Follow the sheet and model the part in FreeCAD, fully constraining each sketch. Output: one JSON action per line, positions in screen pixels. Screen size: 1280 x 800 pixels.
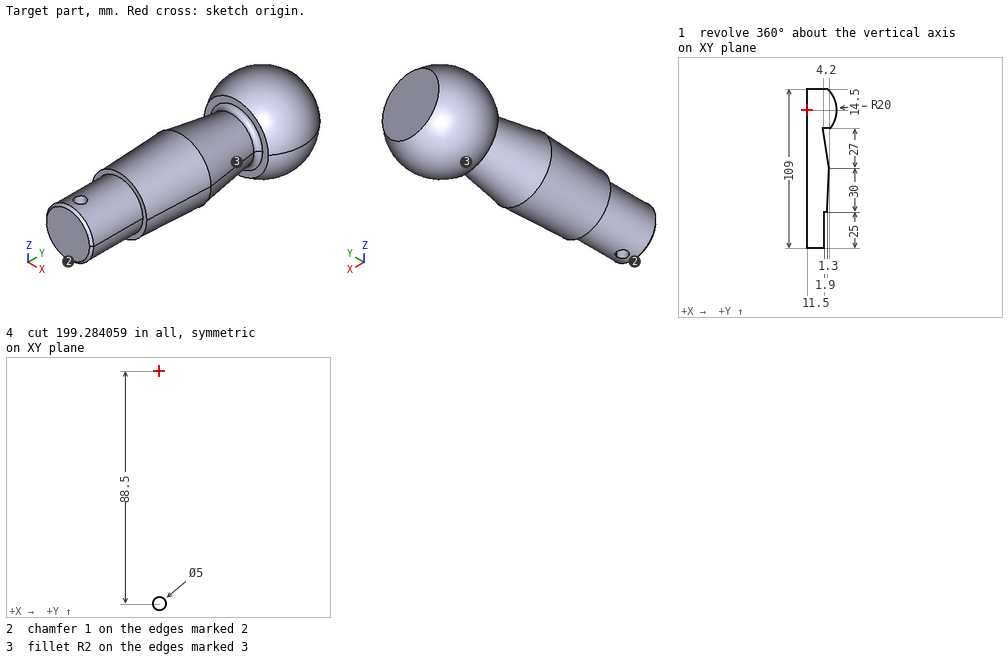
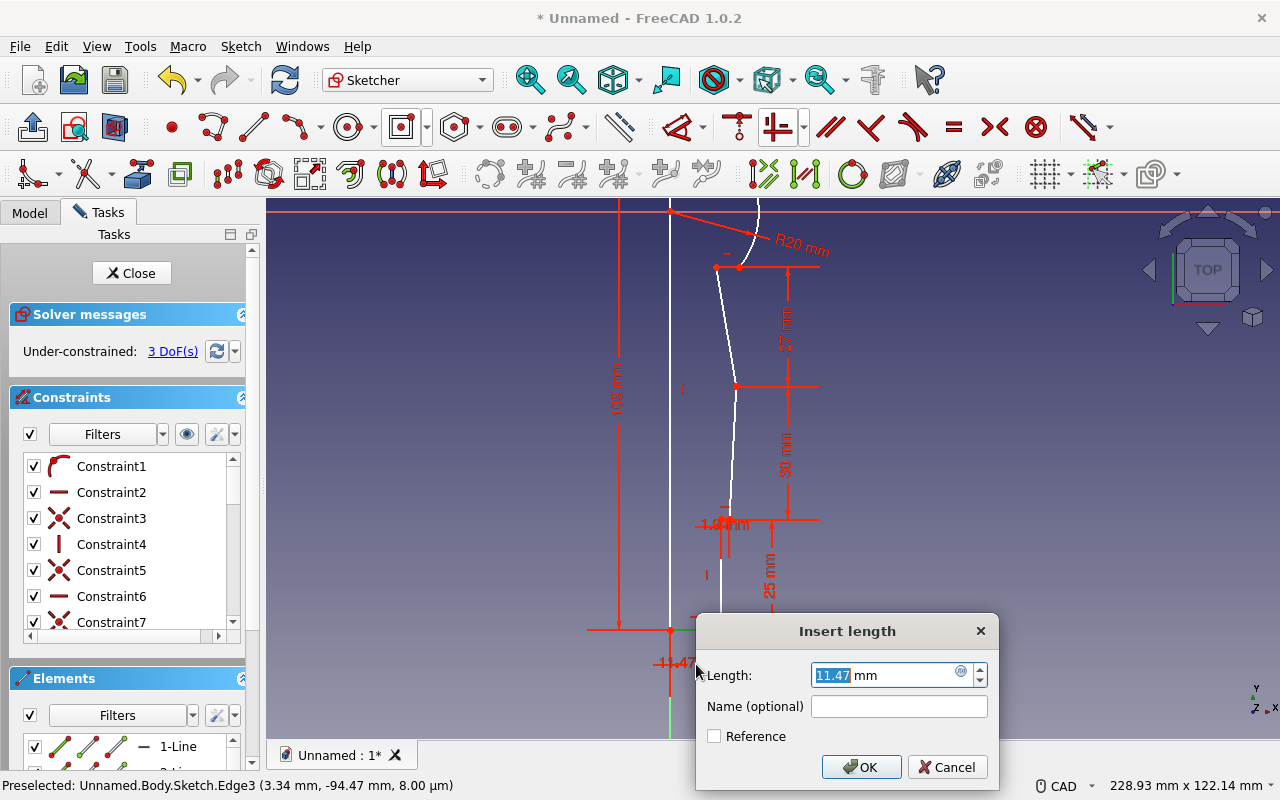
{"action": "type", "text": "11.5"}
{"action": "key", "text": "Return"}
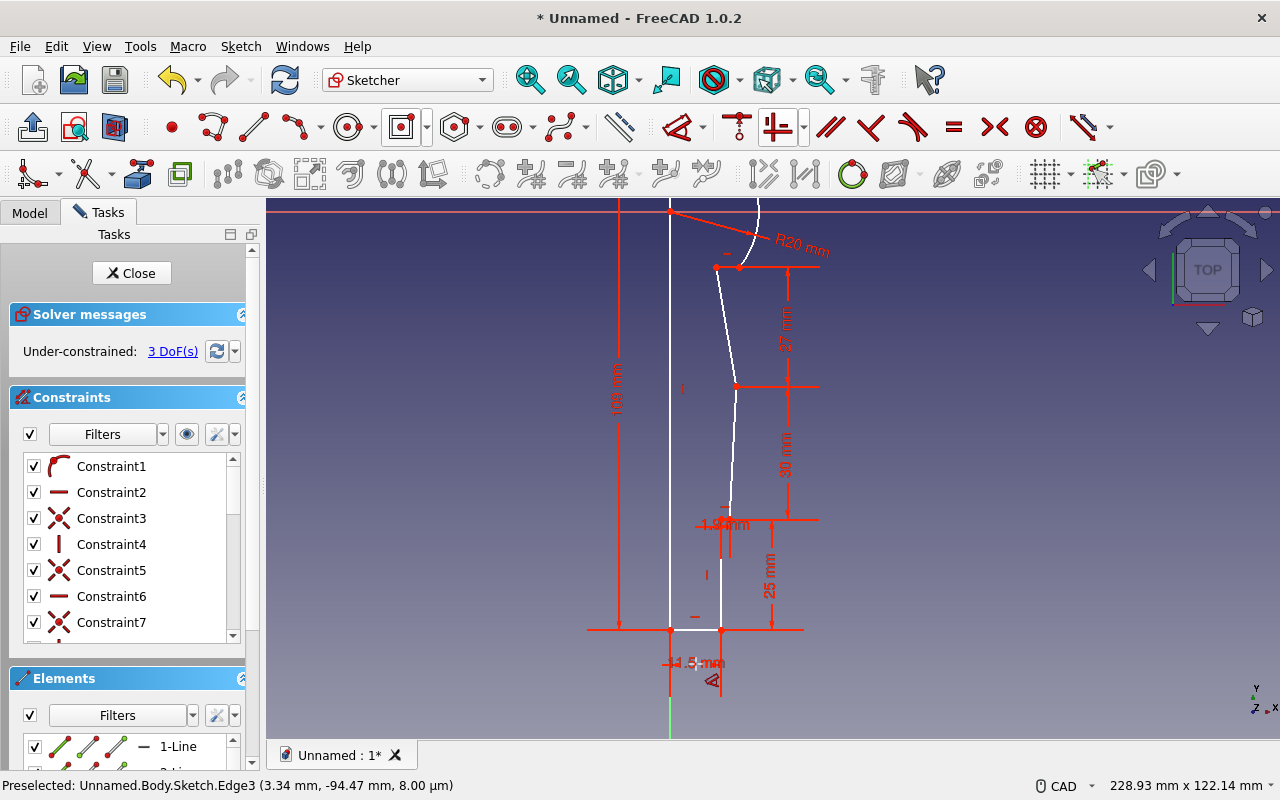
{"action": "scroll", "coordinate": [732, 480], "scroll_direction": "up", "scroll_amount": 10}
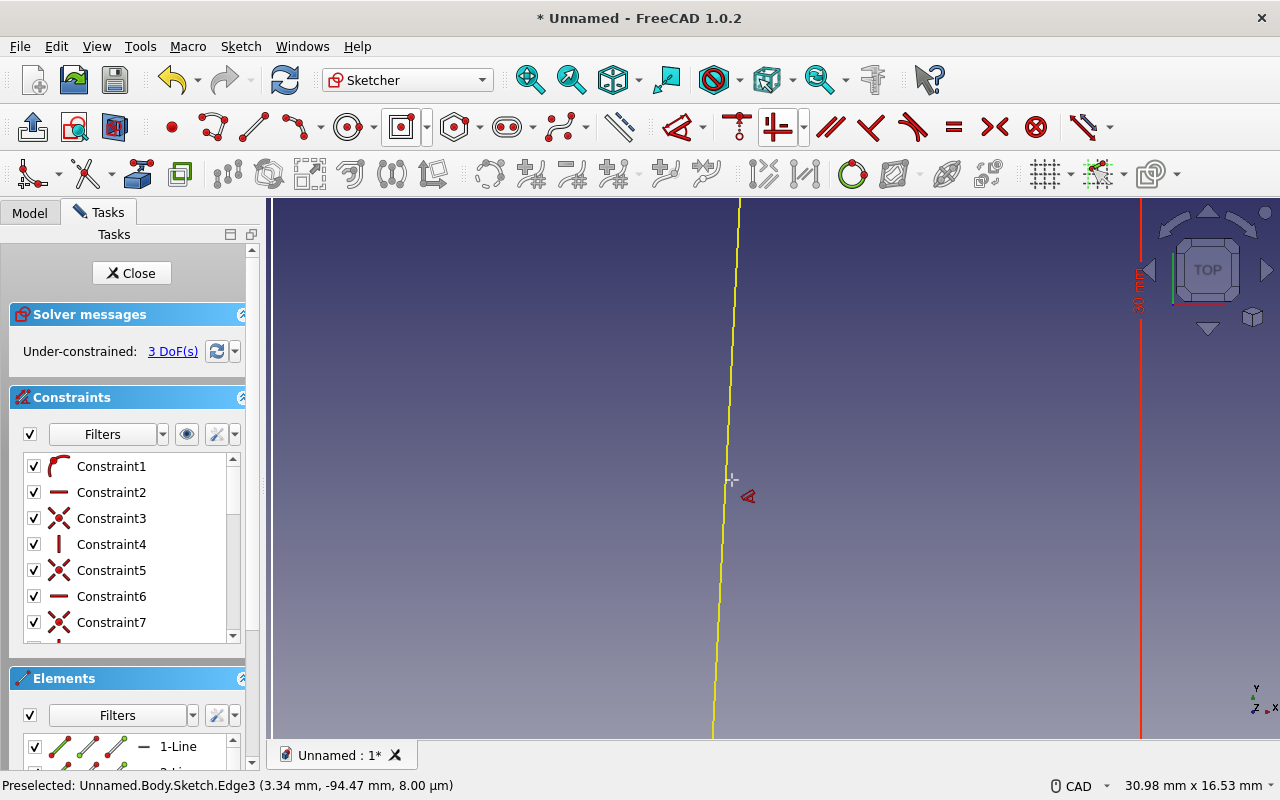
{"action": "left_click", "coordinate": [726, 475]}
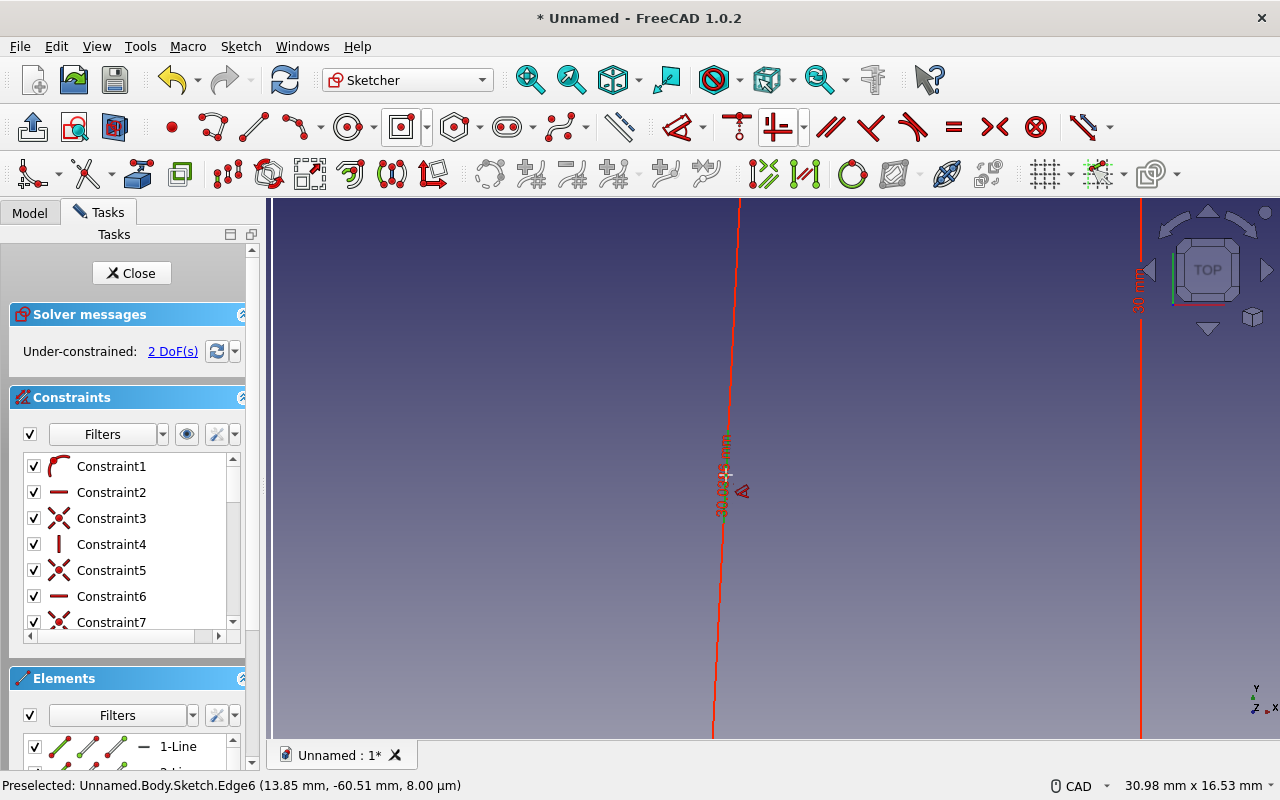
{"action": "key", "text": "Escape"}
{"action": "key", "text": "Escape"}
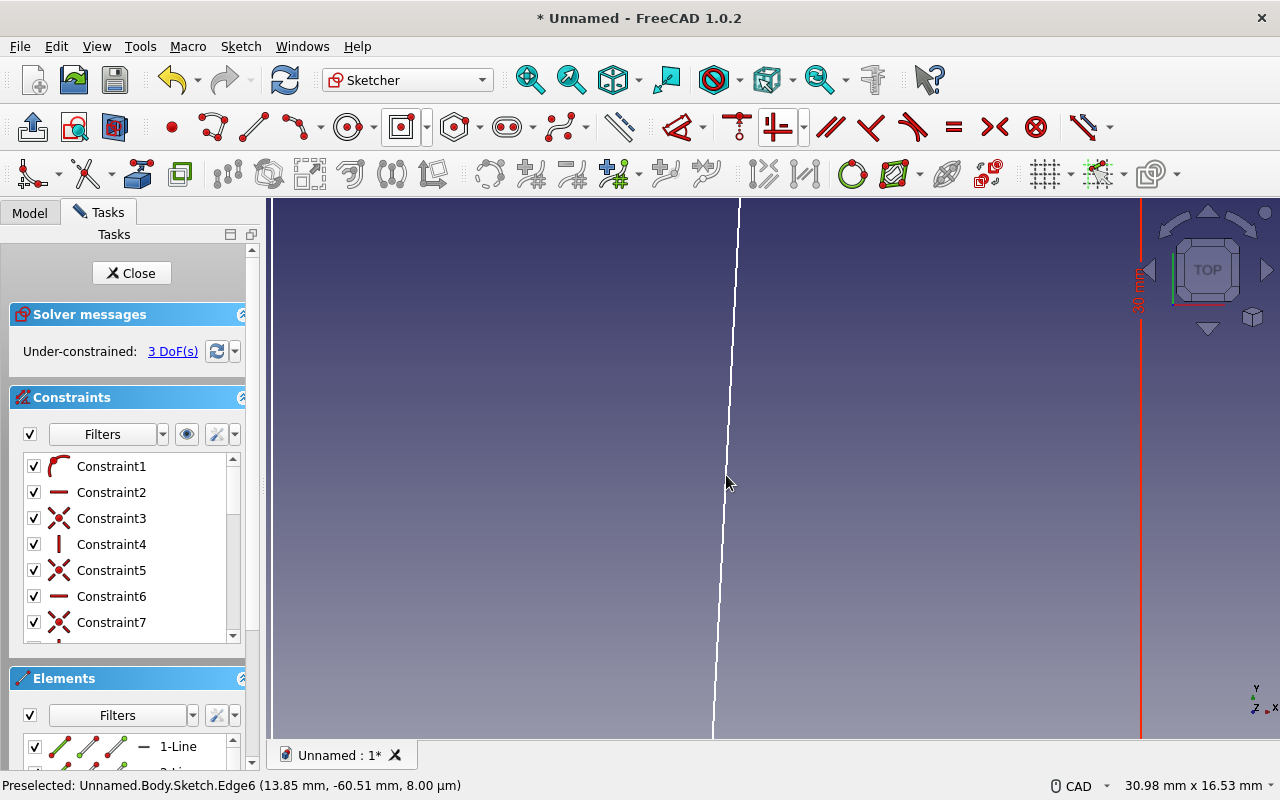
{"action": "left_click", "coordinate": [726, 475]}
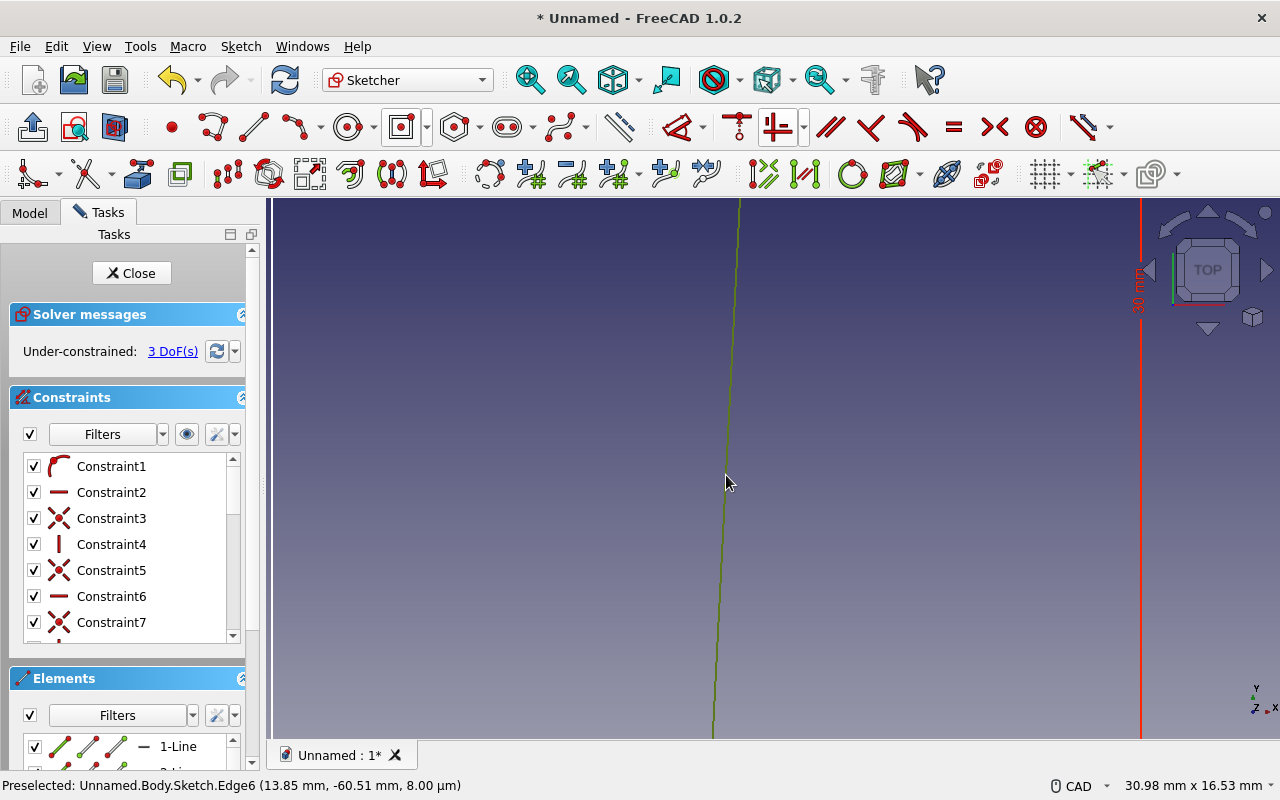
{"action": "left_click", "coordinate": [702, 128]}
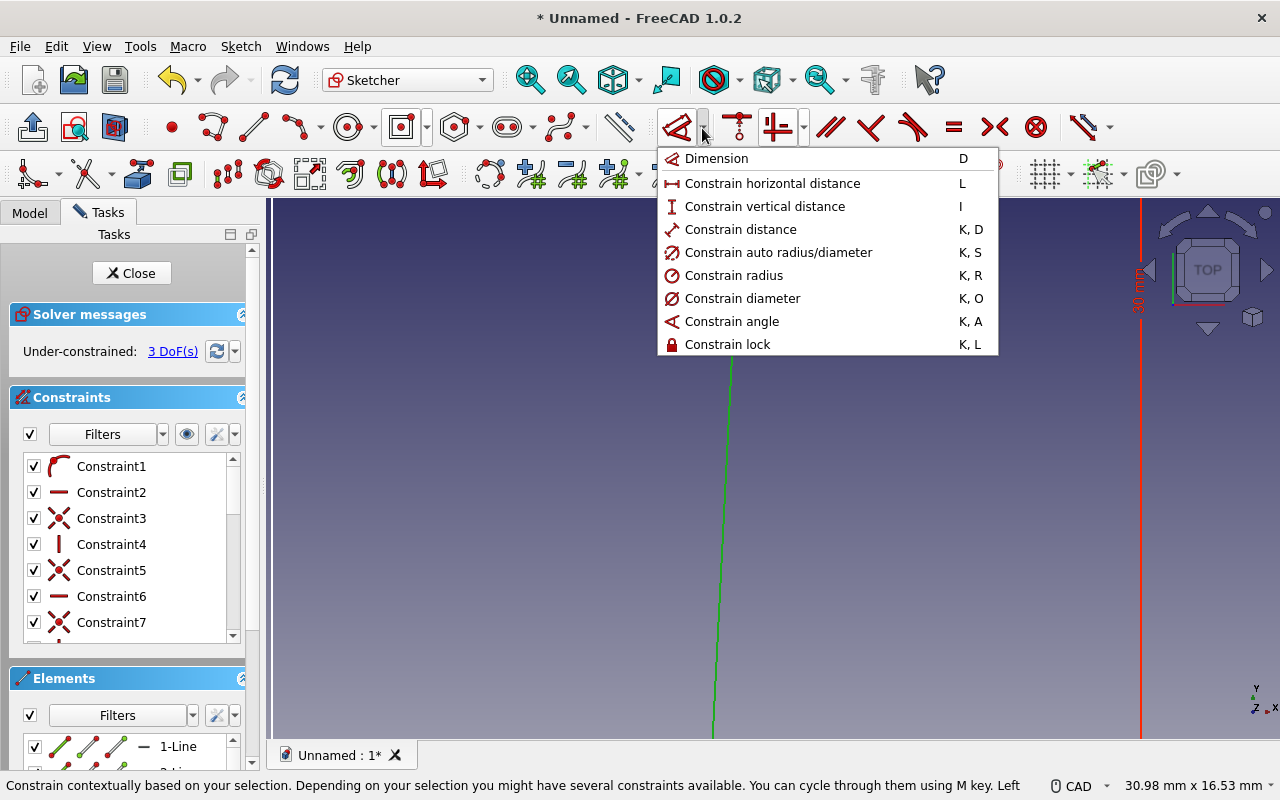
{"action": "left_click", "coordinate": [828, 184]}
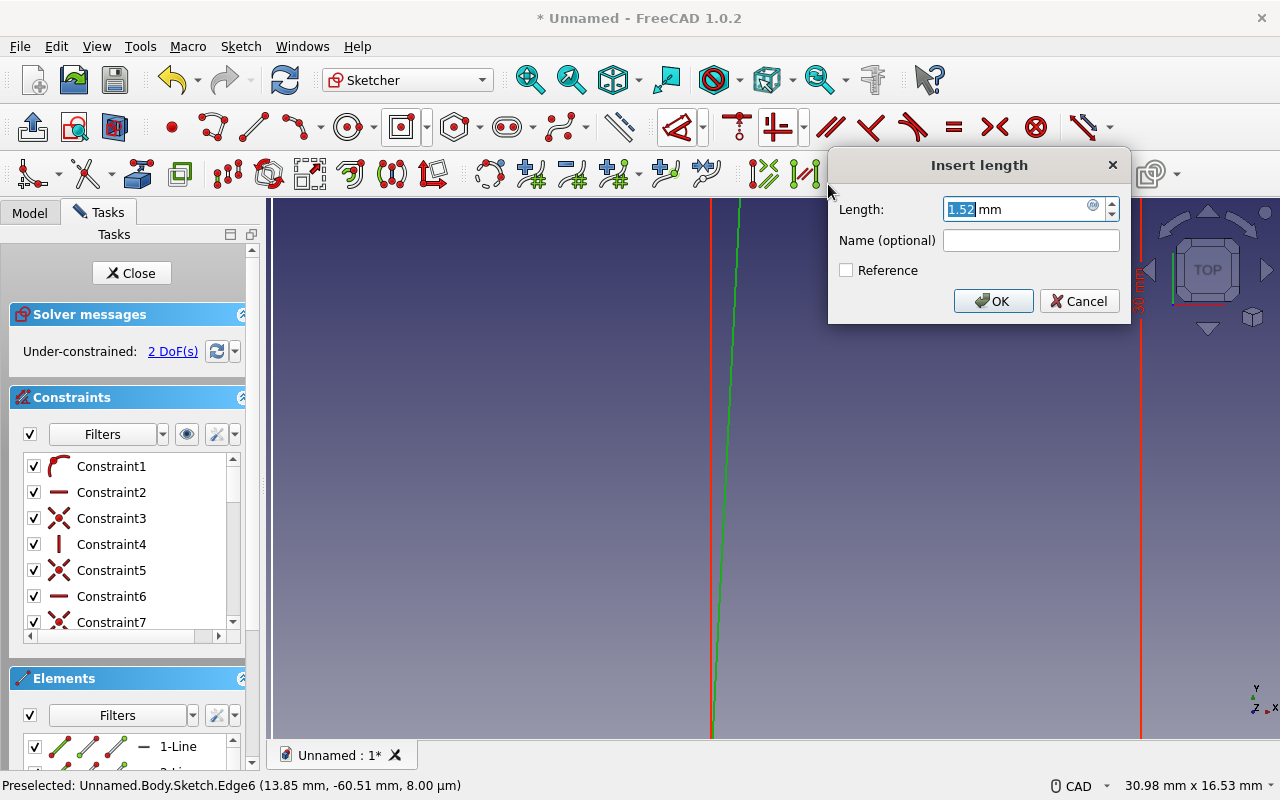
{"action": "type", "text": "1.3"}
{"action": "key", "text": "Return"}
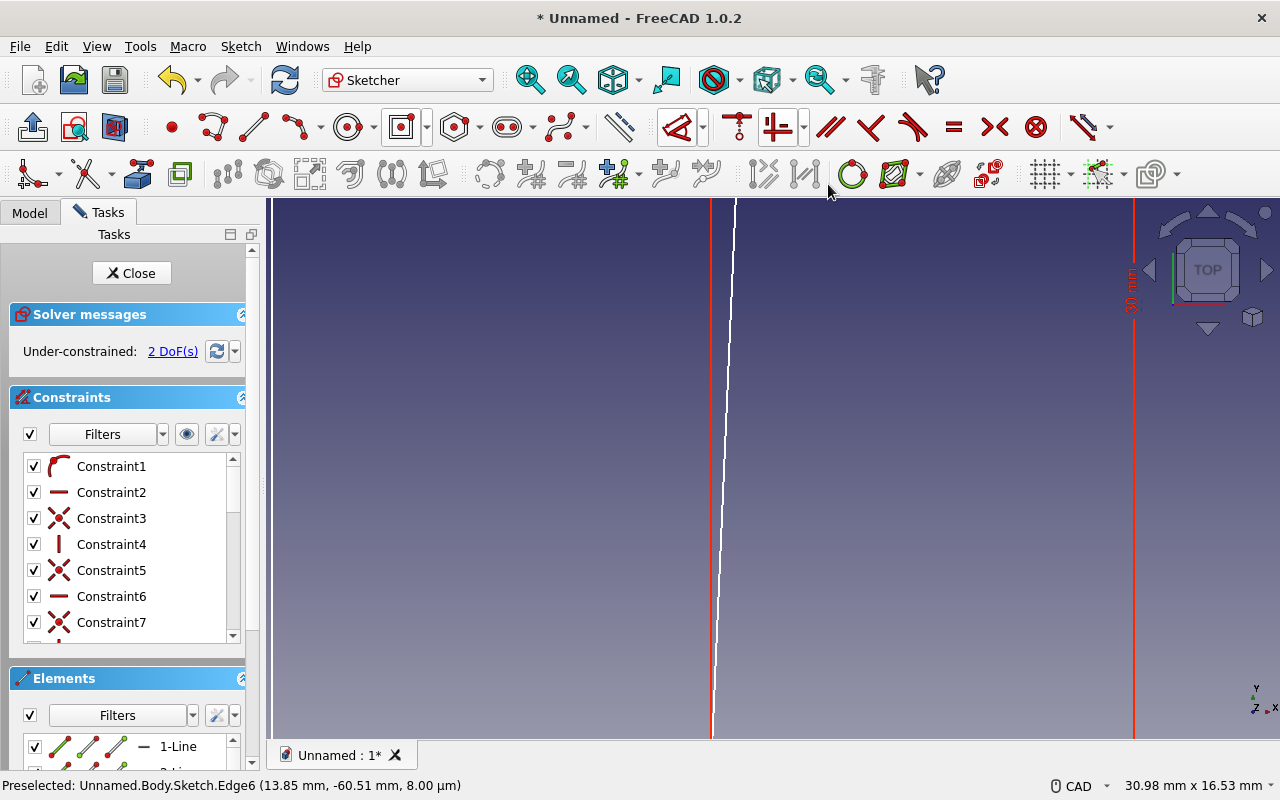
{"action": "scroll", "coordinate": [715, 535], "scroll_direction": "down", "scroll_amount": 12}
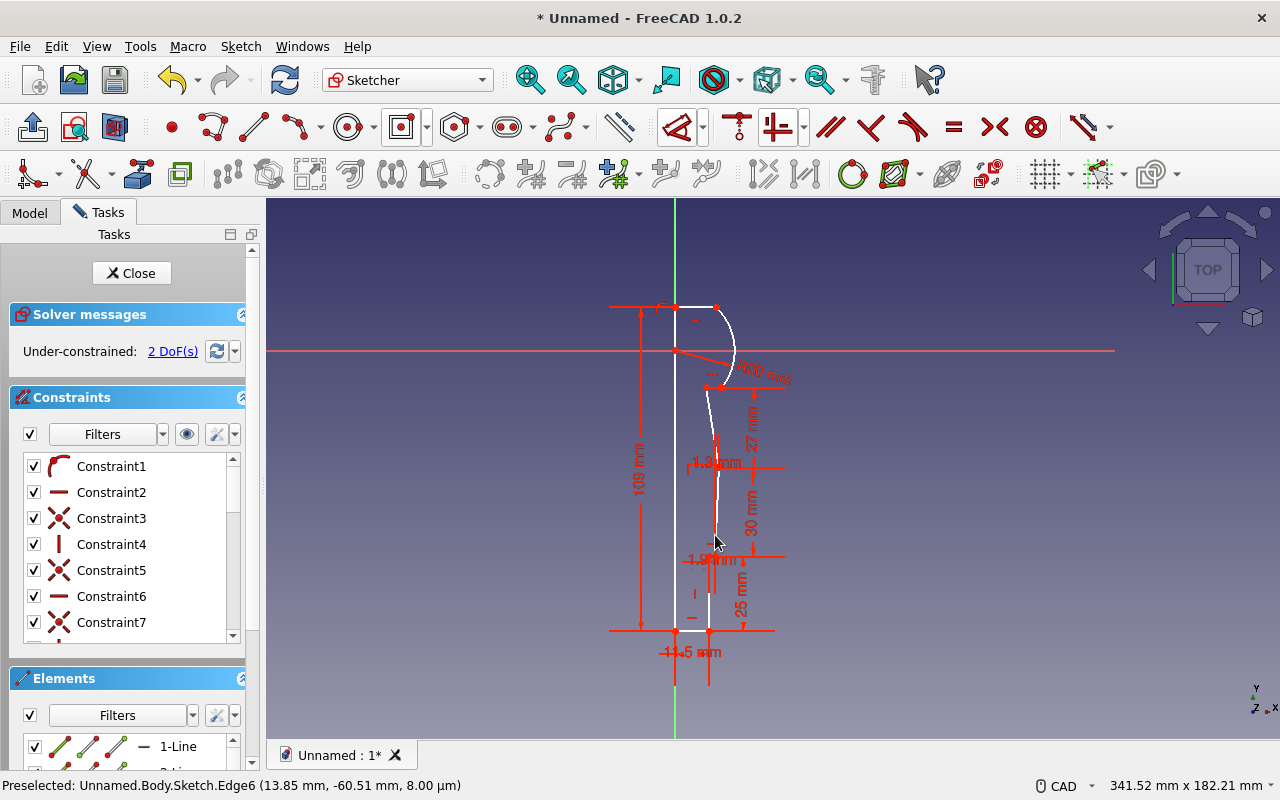
{"action": "scroll", "coordinate": [715, 444], "scroll_direction": "up", "scroll_amount": 6}